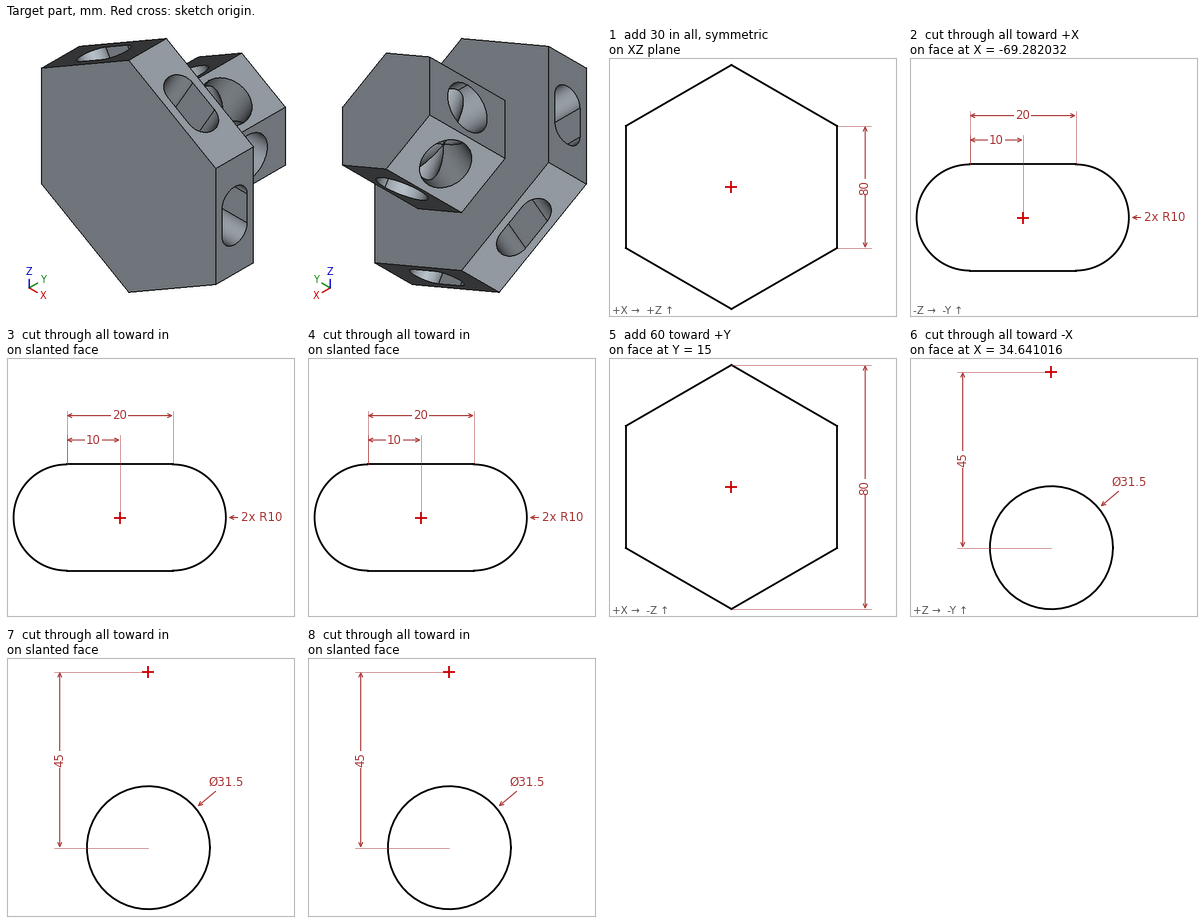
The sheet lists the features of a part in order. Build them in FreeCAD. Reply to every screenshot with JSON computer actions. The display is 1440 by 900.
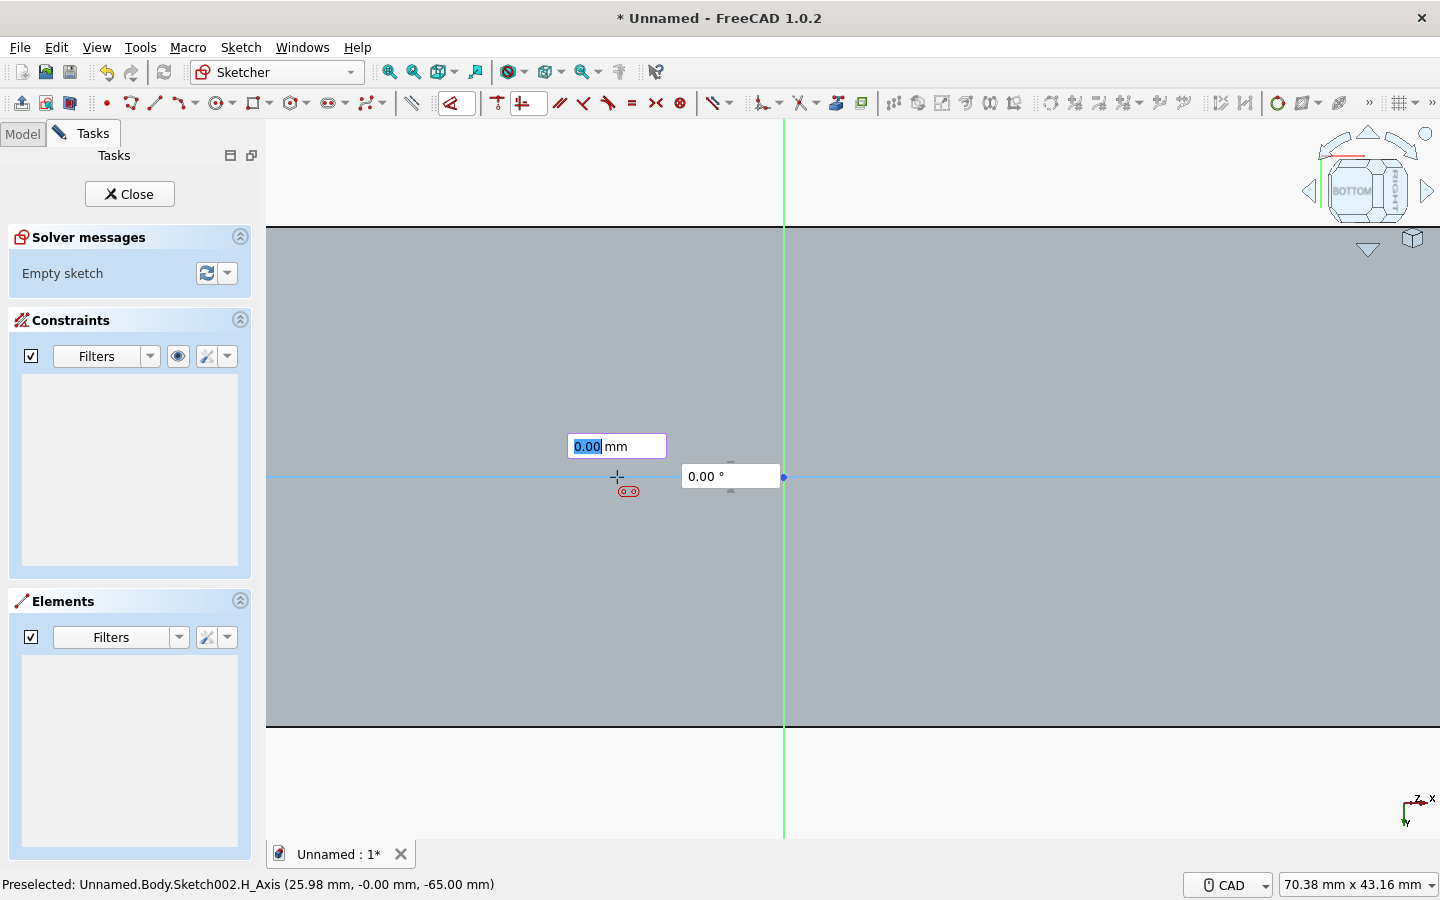
{"action": "left_click", "coordinate": [951, 468]}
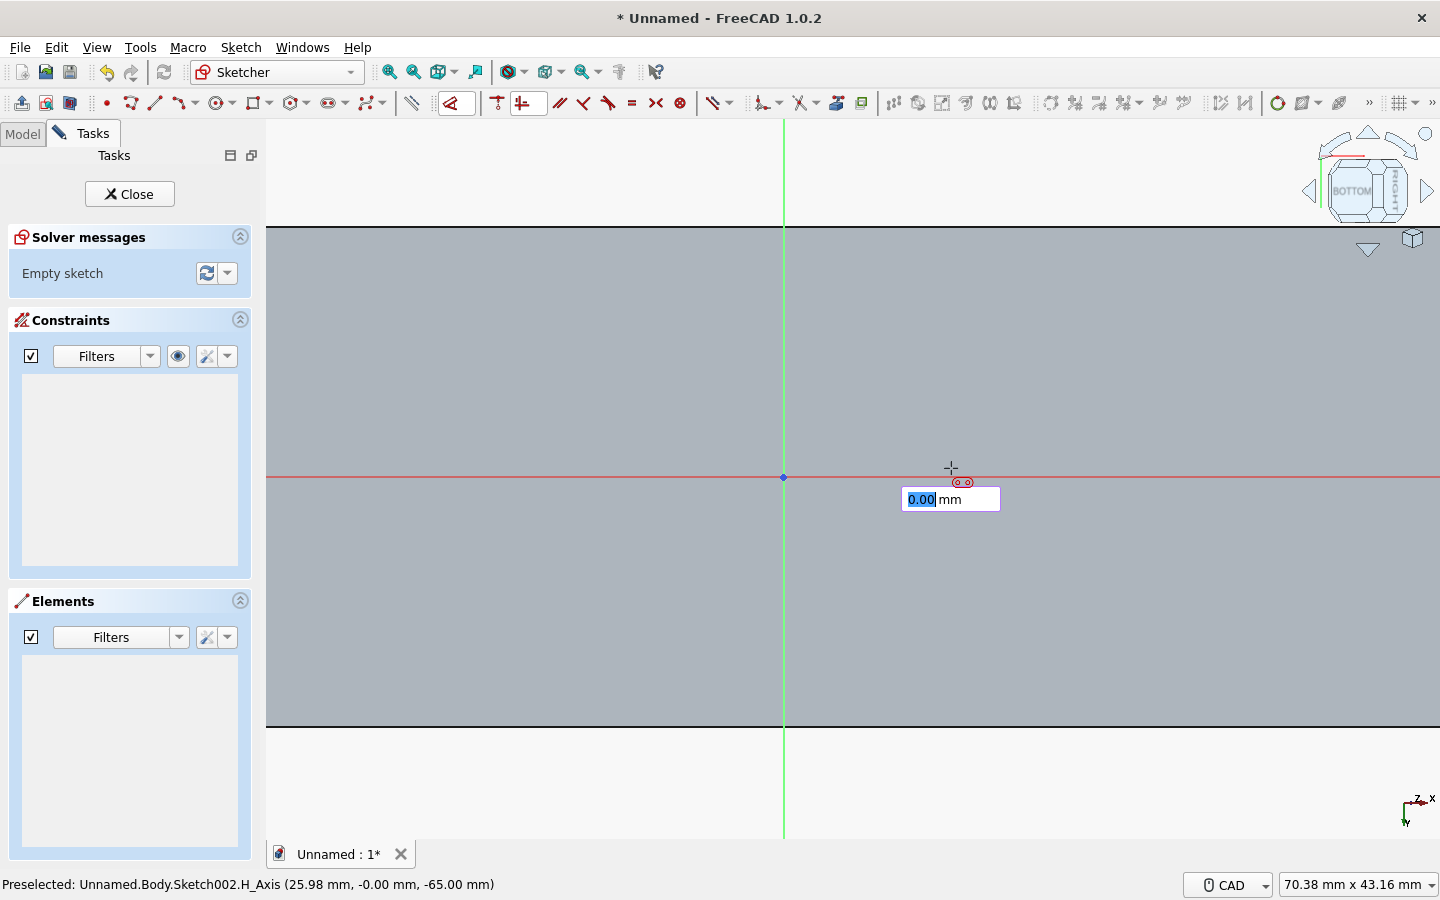
{"action": "left_click", "coordinate": [734, 644]}
{"action": "key", "text": "Escape"}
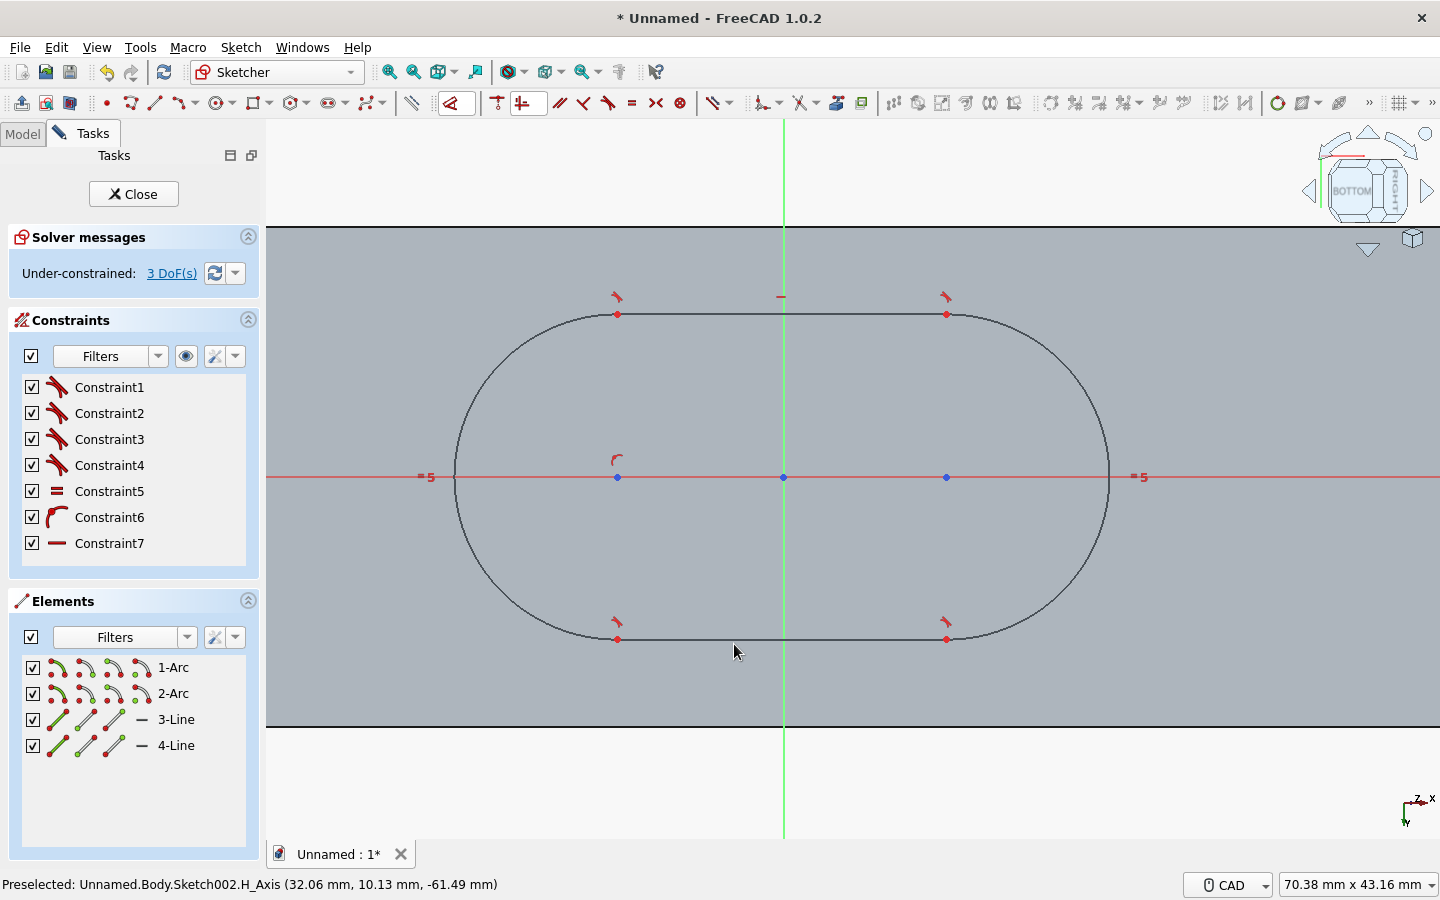
{"action": "left_click", "coordinate": [486, 381]}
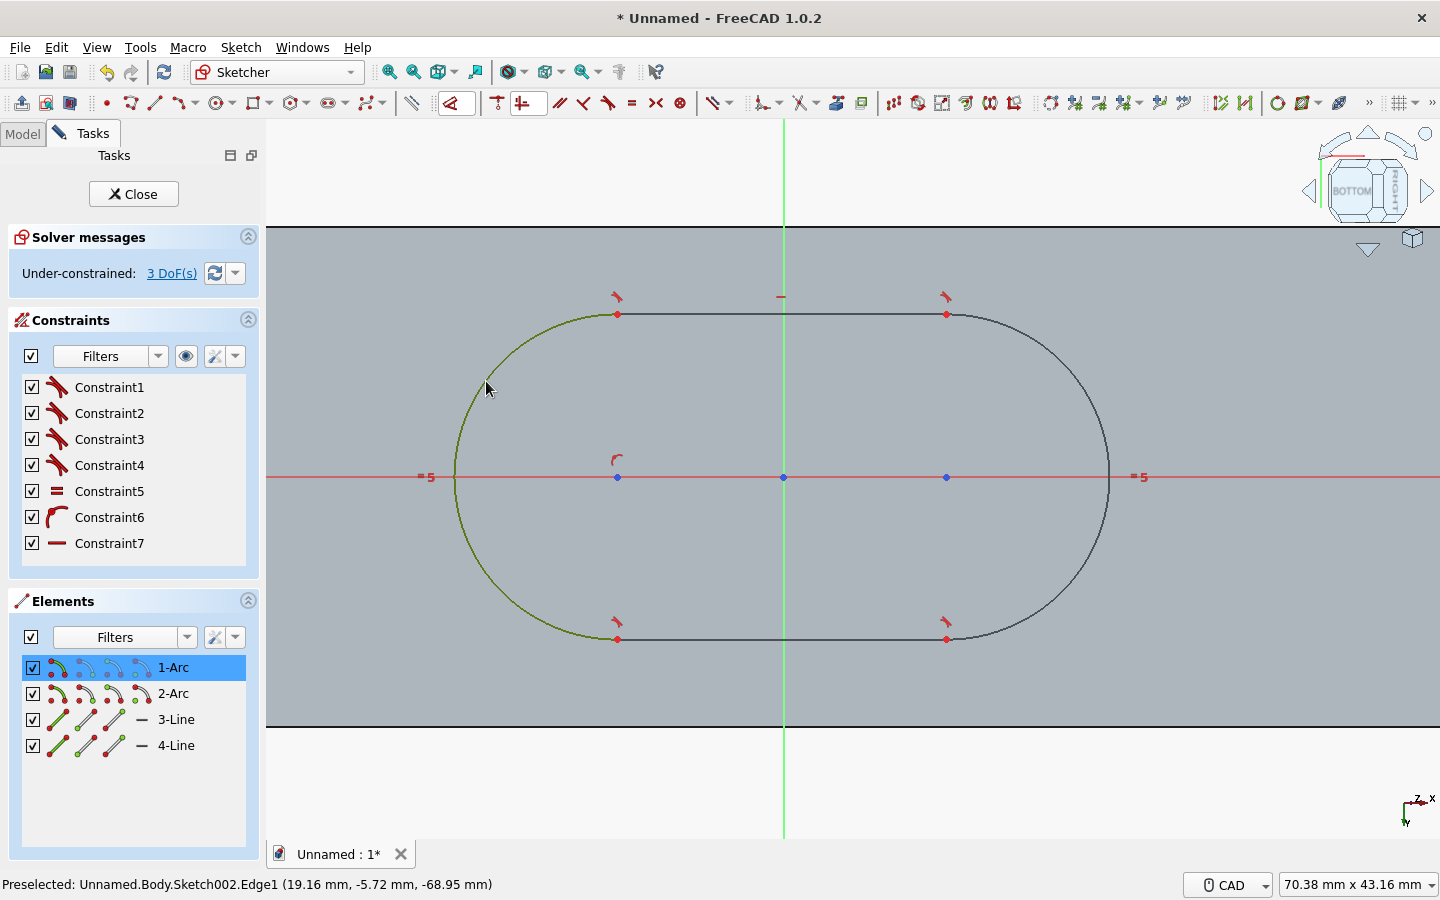
{"action": "left_click", "coordinate": [470, 104]}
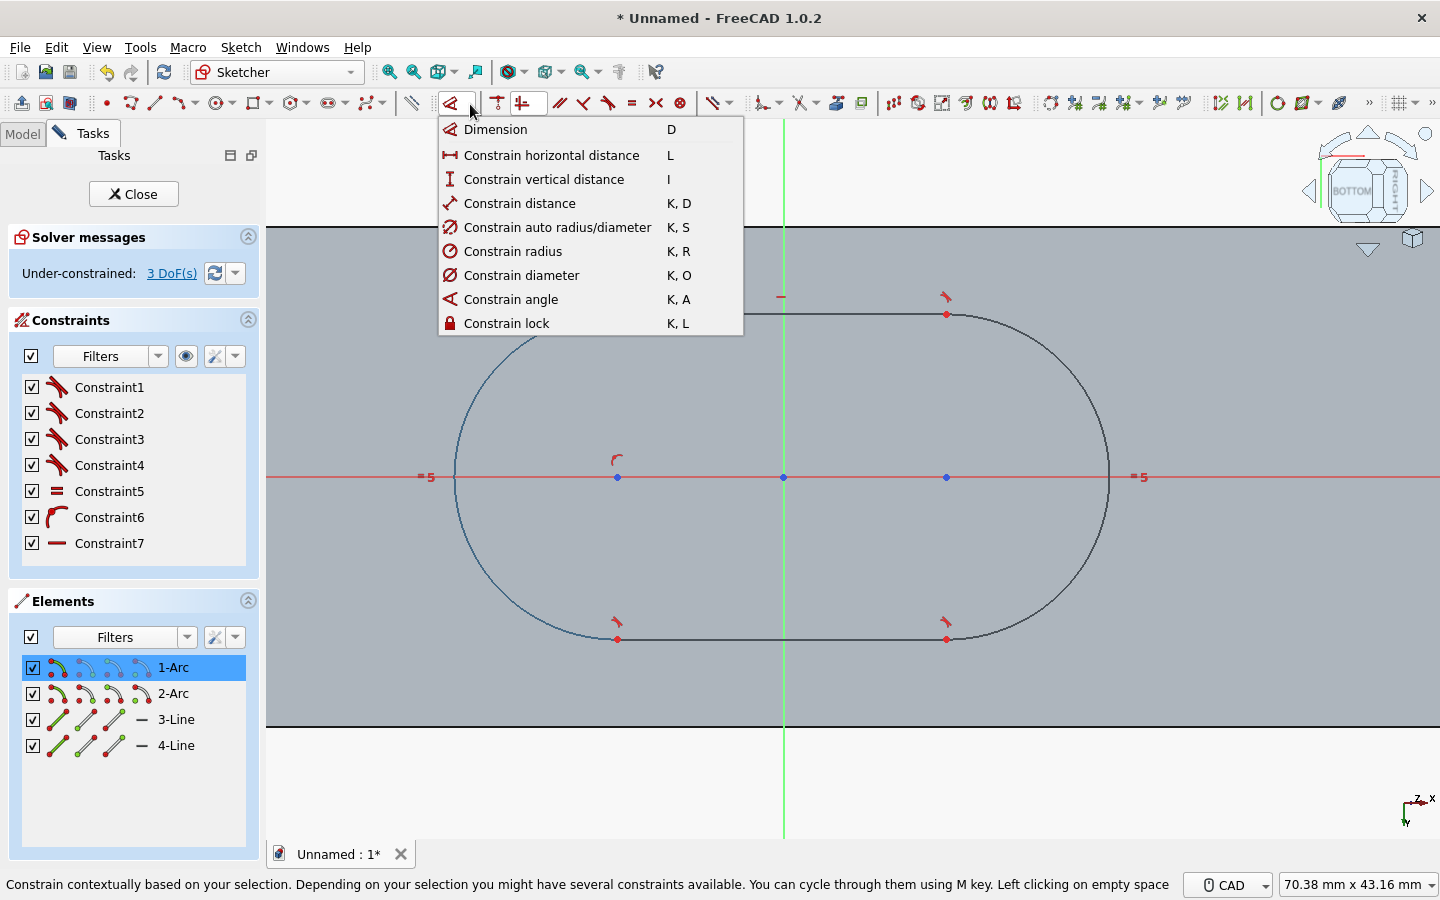
{"action": "left_click", "coordinate": [591, 251]}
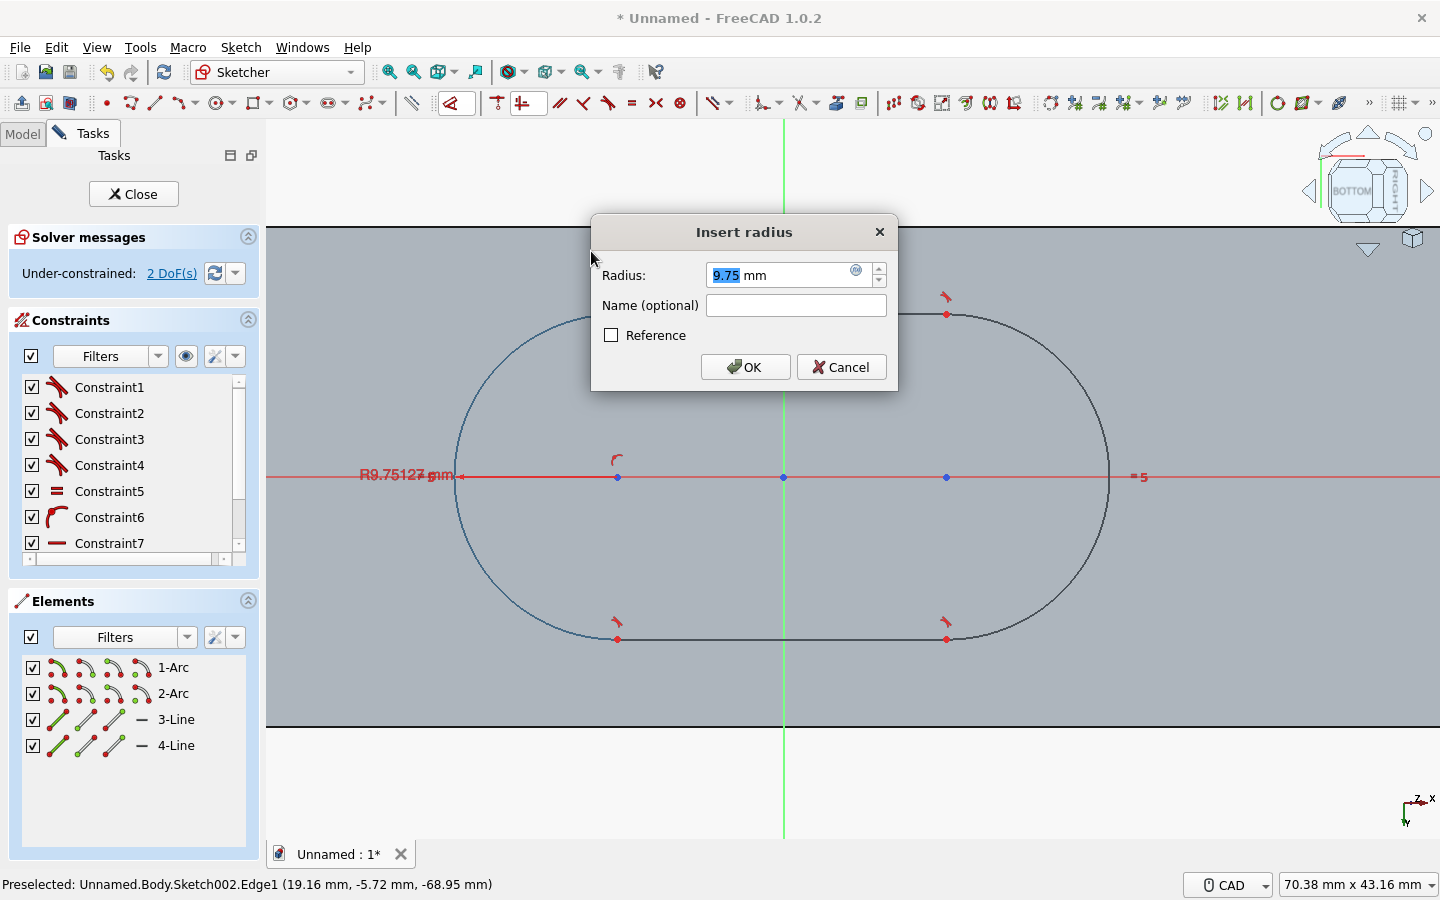
{"action": "type", "text": "10"}
{"action": "key", "text": "Return"}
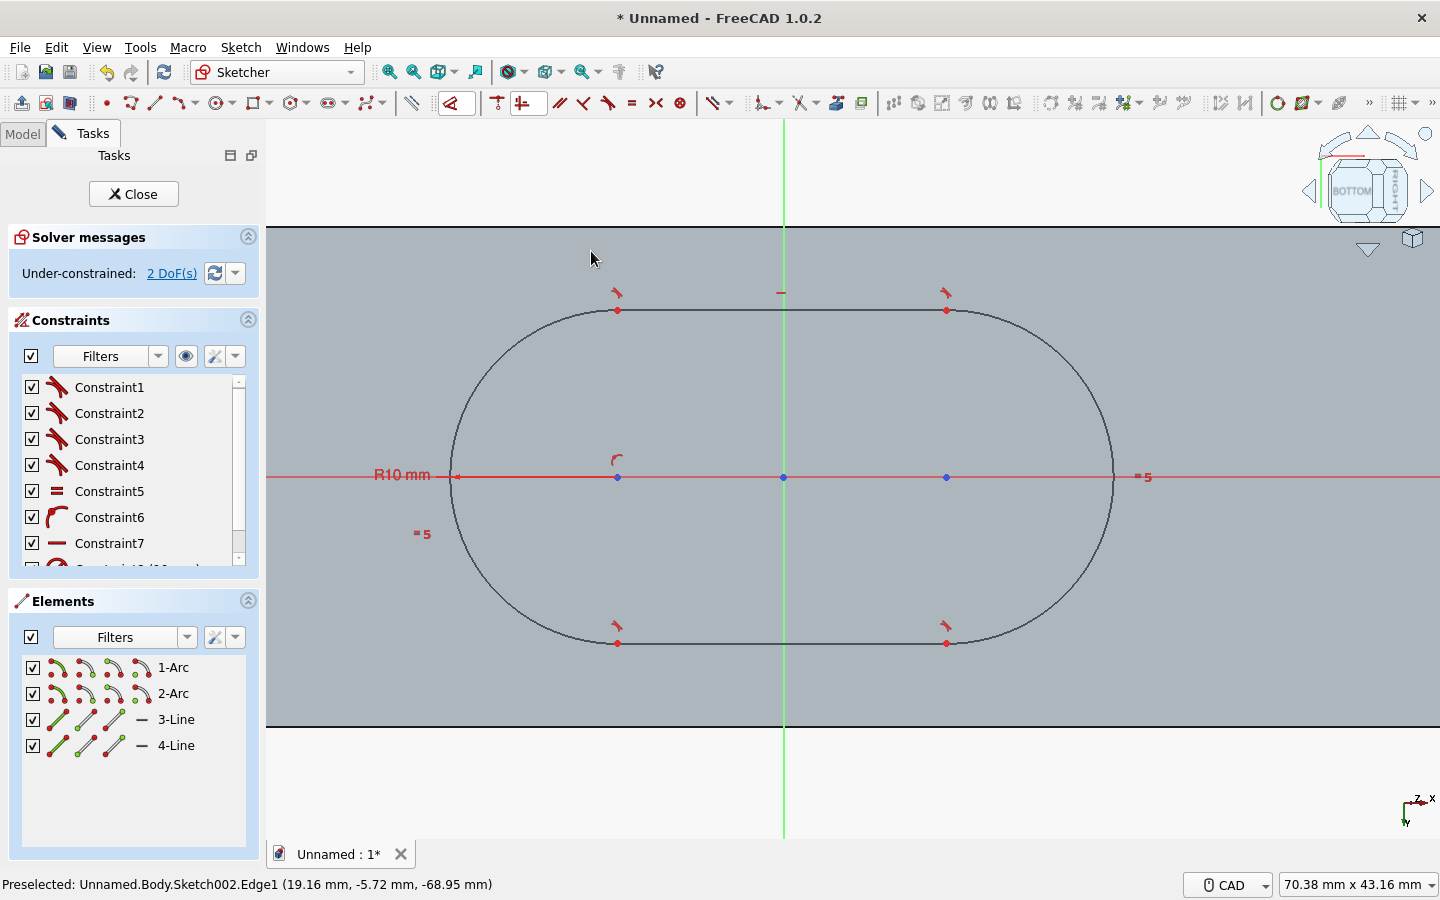
{"action": "left_click", "coordinate": [716, 310]}